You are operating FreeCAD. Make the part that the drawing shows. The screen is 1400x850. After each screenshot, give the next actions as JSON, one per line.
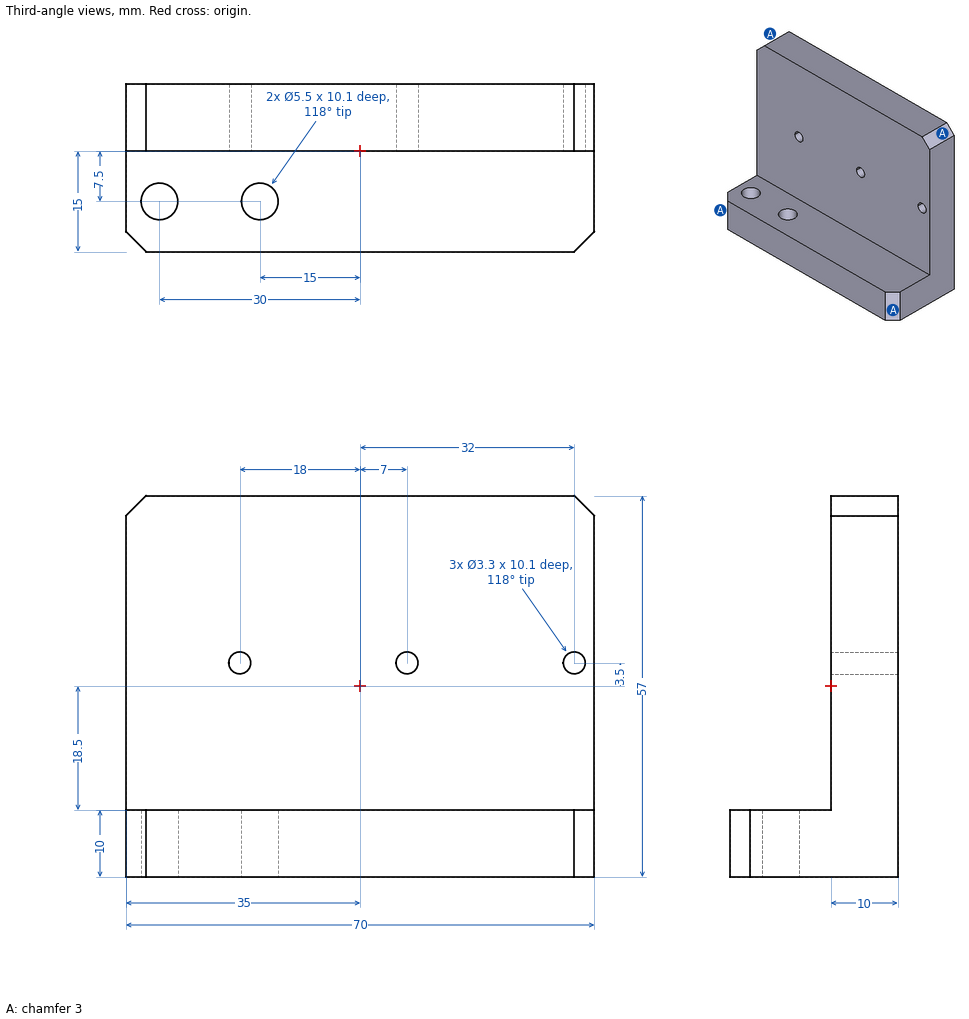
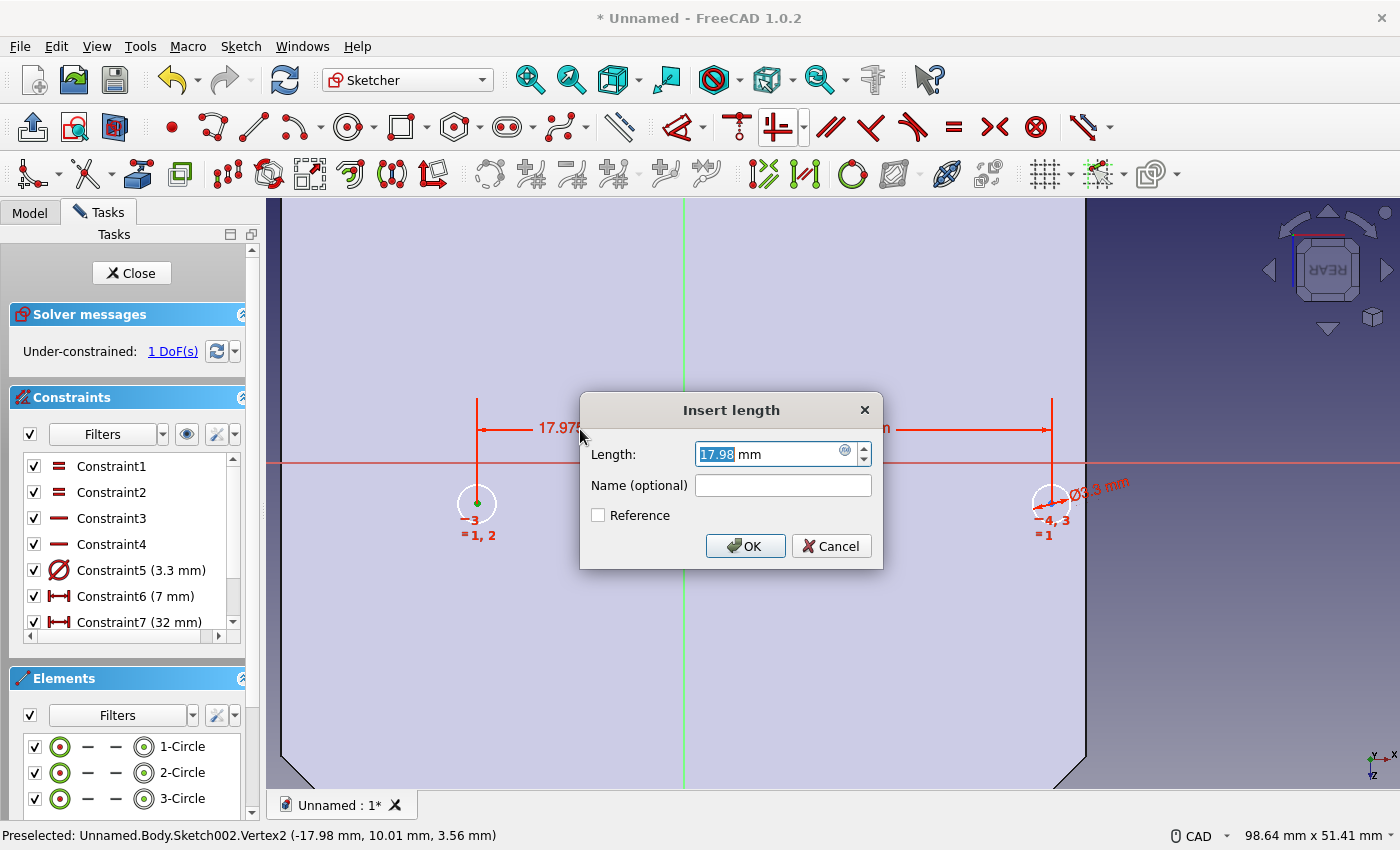
{"action": "type", "text": "18"}
{"action": "key", "text": "Return"}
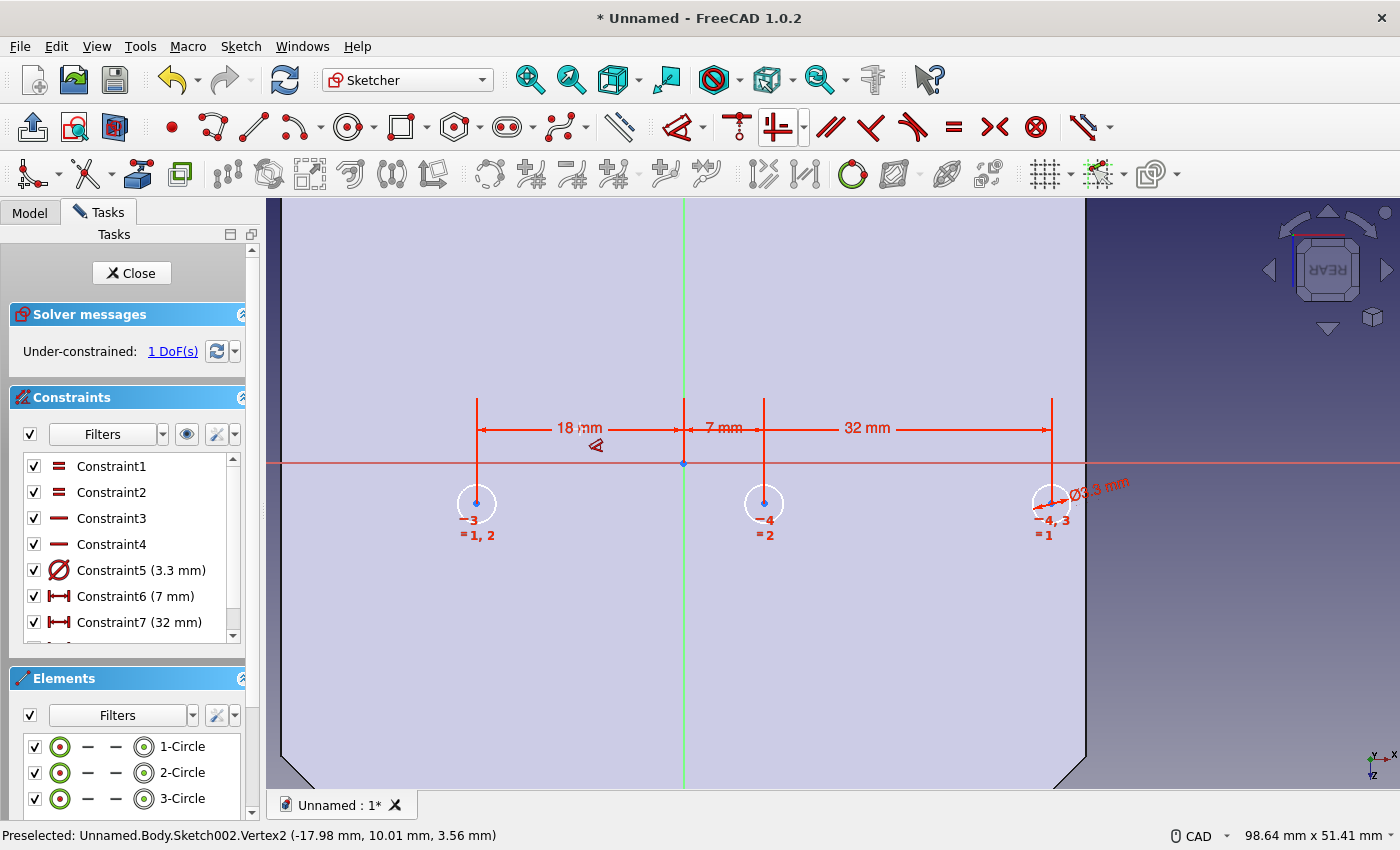
{"action": "left_click", "coordinate": [1052, 504]}
{"action": "left_click", "coordinate": [650, 484]}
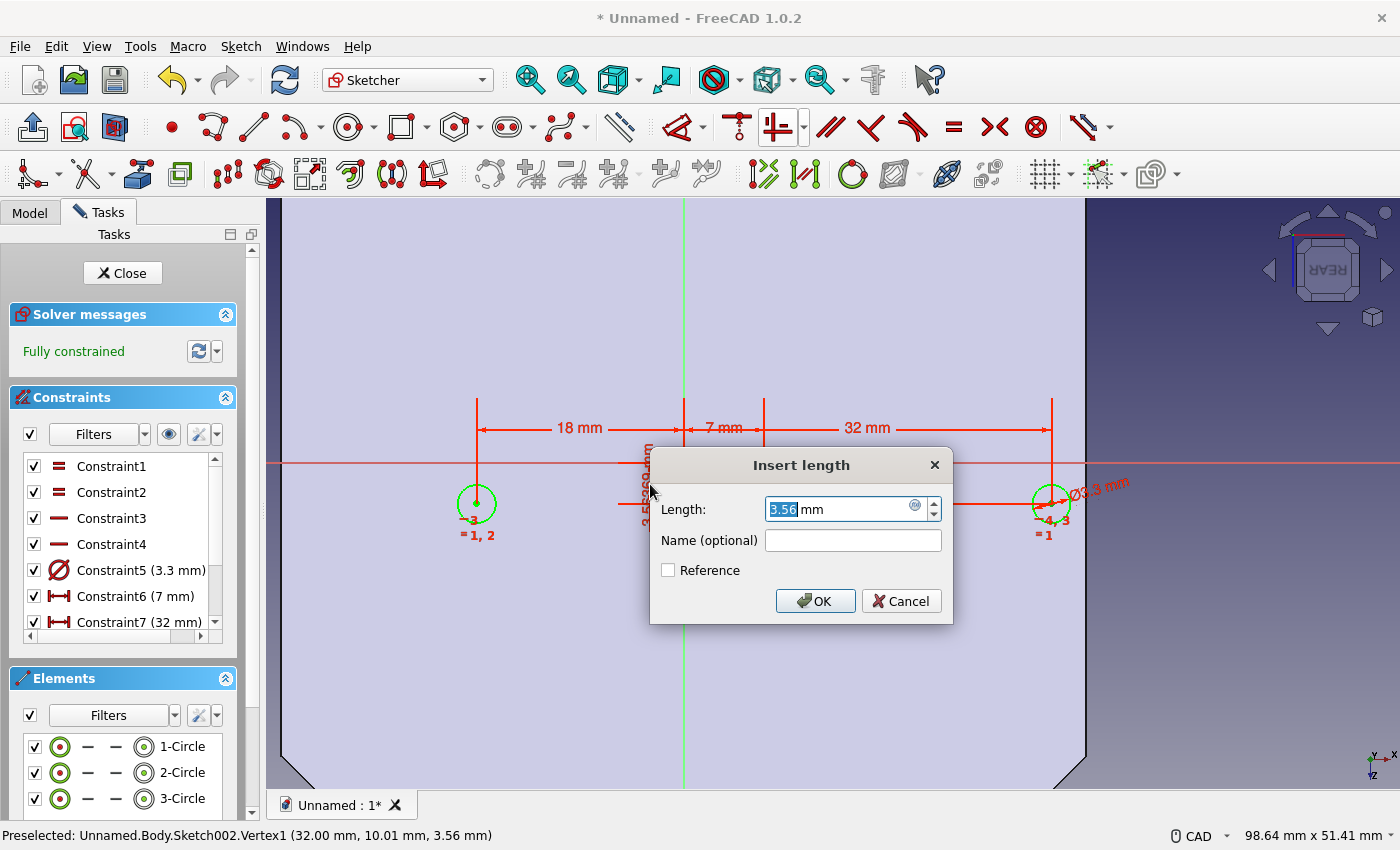
{"action": "type", "text": "3.5"}
{"action": "key", "text": "Return"}
{"action": "key", "text": "Escape"}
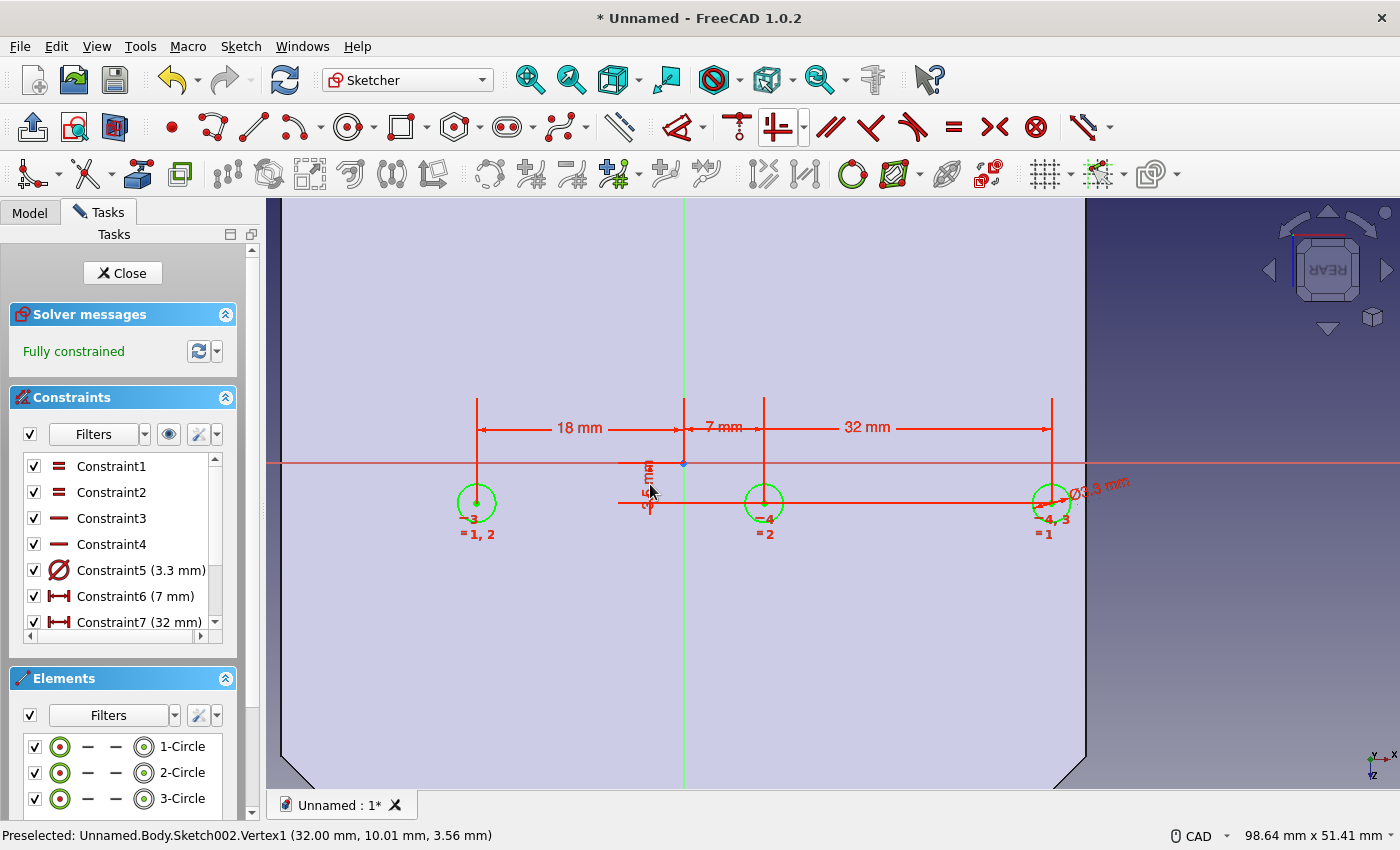
{"action": "left_click", "coordinate": [123, 273]}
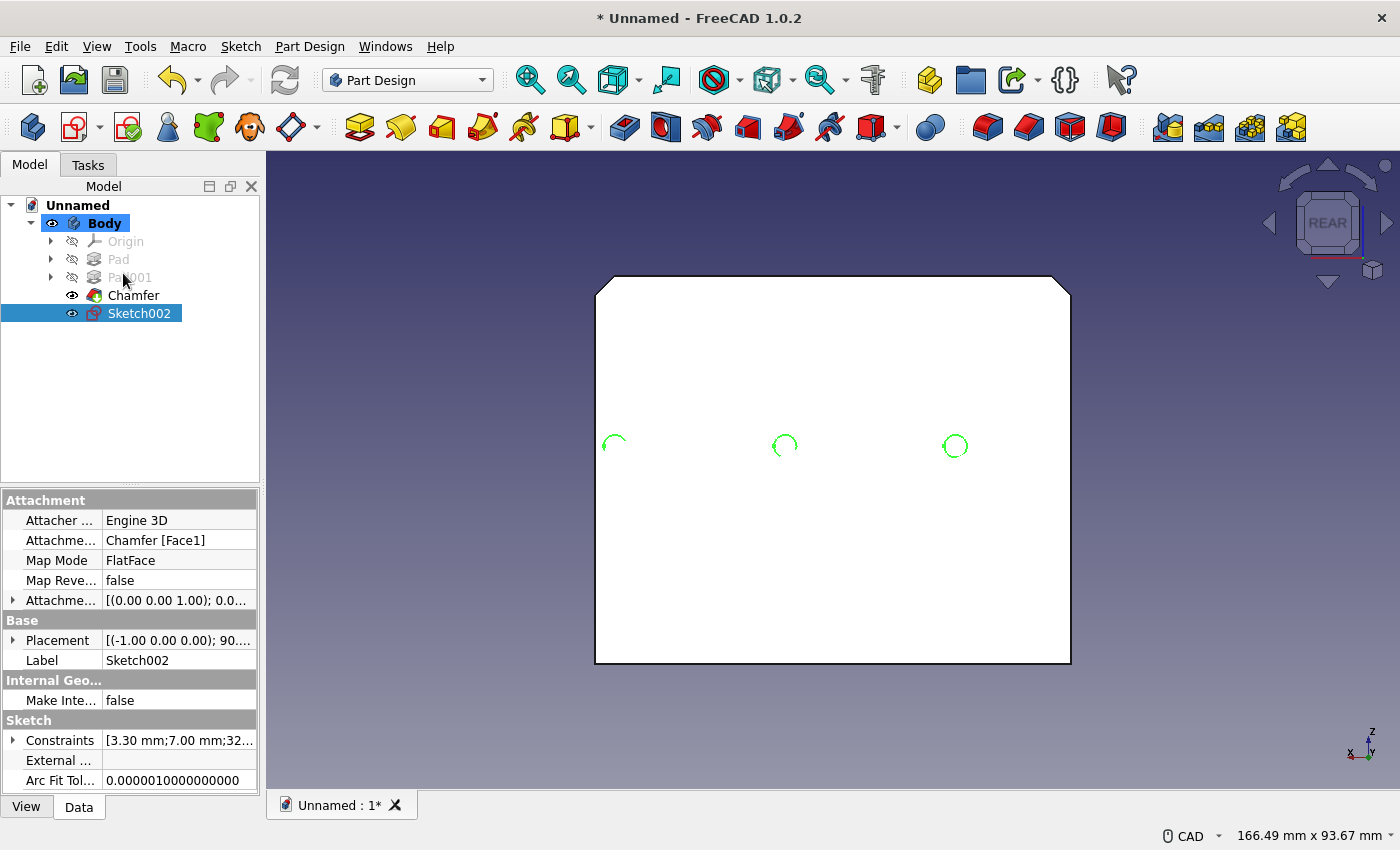
{"action": "left_click", "coordinate": [666, 128]}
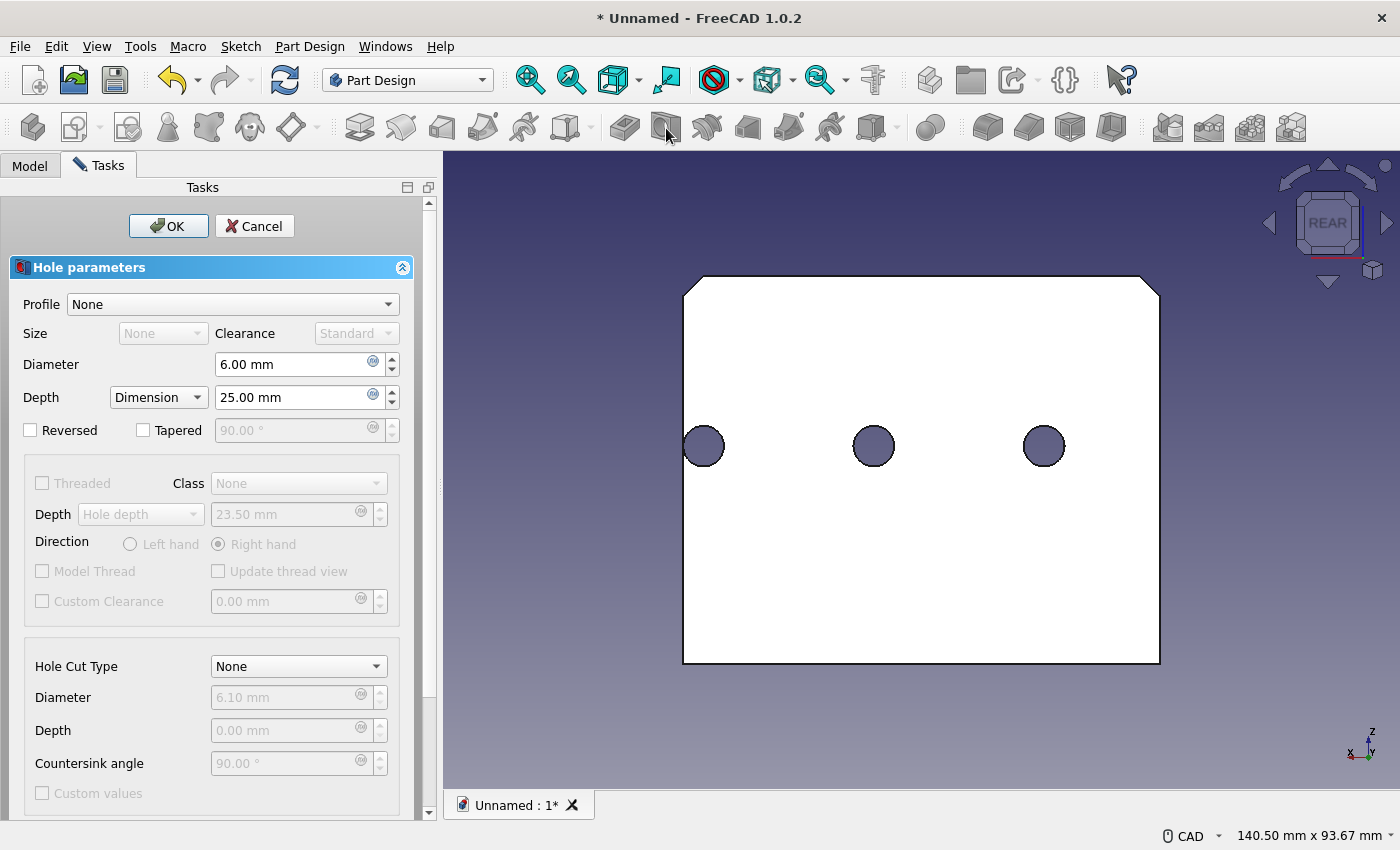
{"action": "triple_click", "coordinate": [300, 364]}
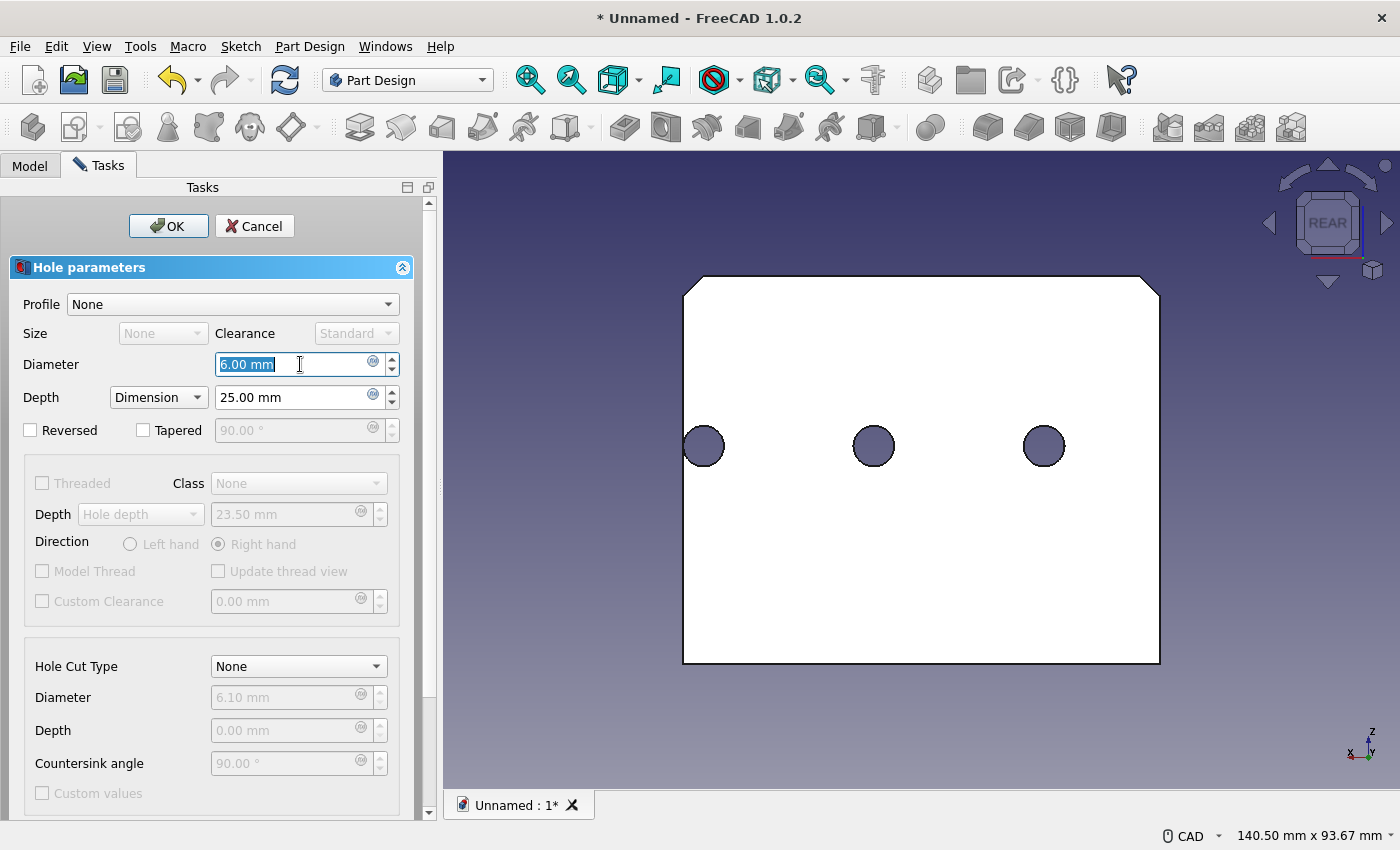
{"action": "type", "text": "3.3"}
{"action": "key", "text": "Tab"}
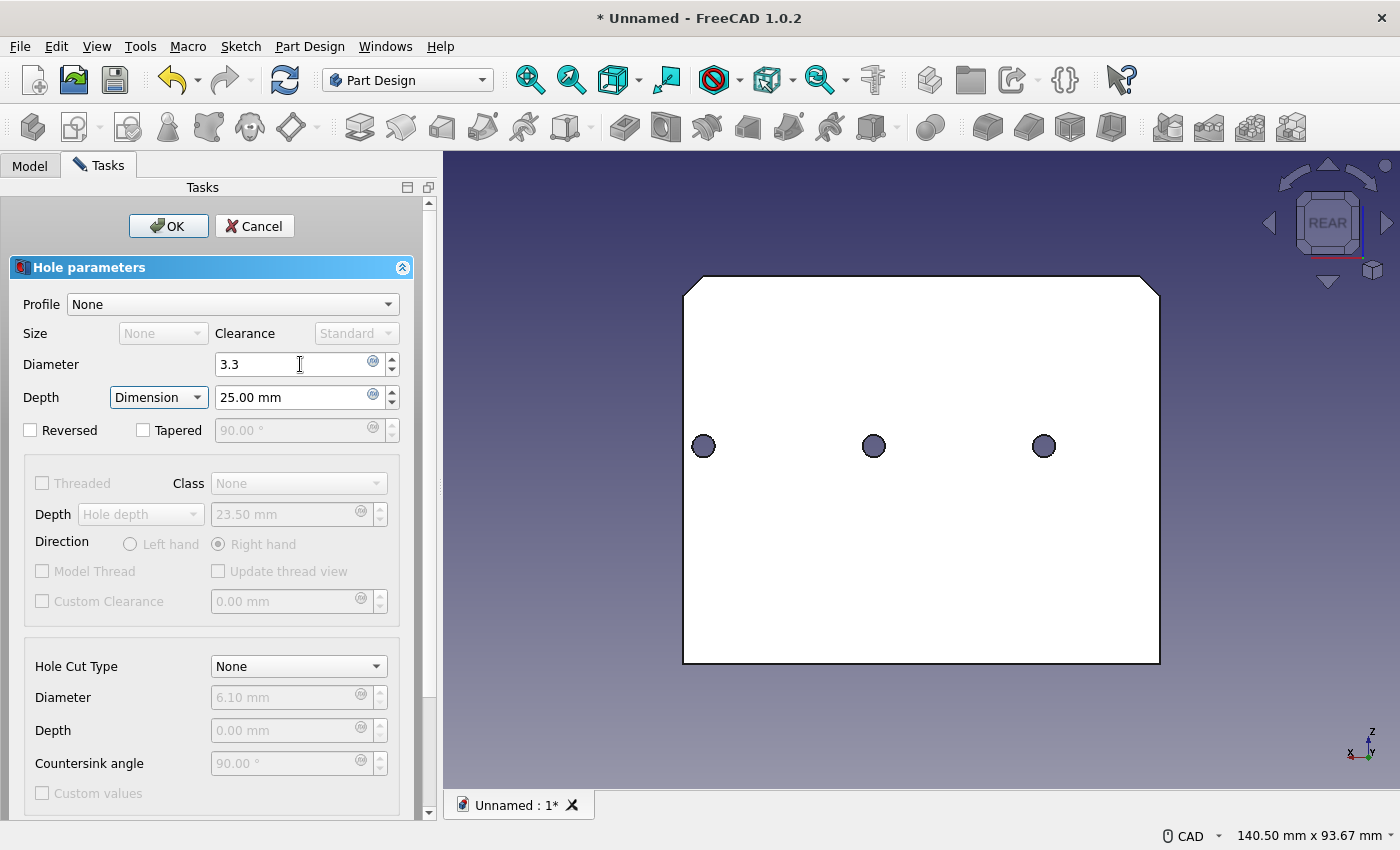
{"action": "triple_click", "coordinate": [300, 398]}